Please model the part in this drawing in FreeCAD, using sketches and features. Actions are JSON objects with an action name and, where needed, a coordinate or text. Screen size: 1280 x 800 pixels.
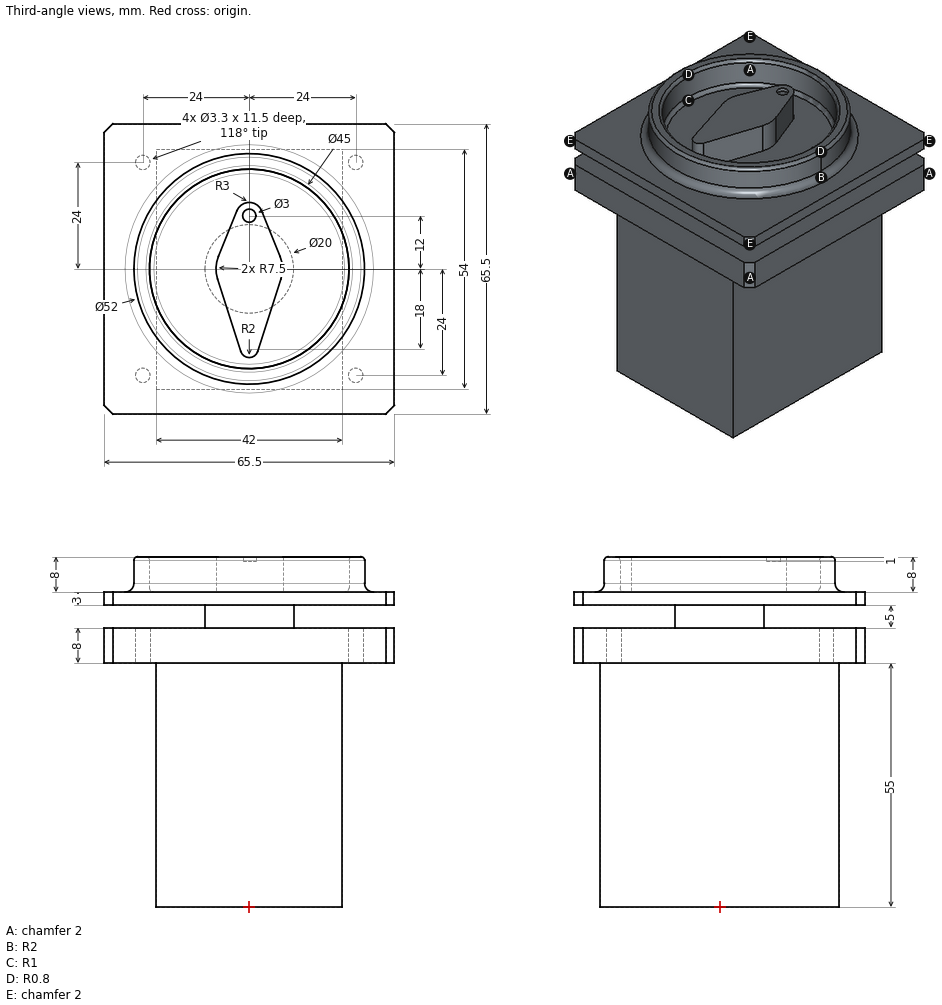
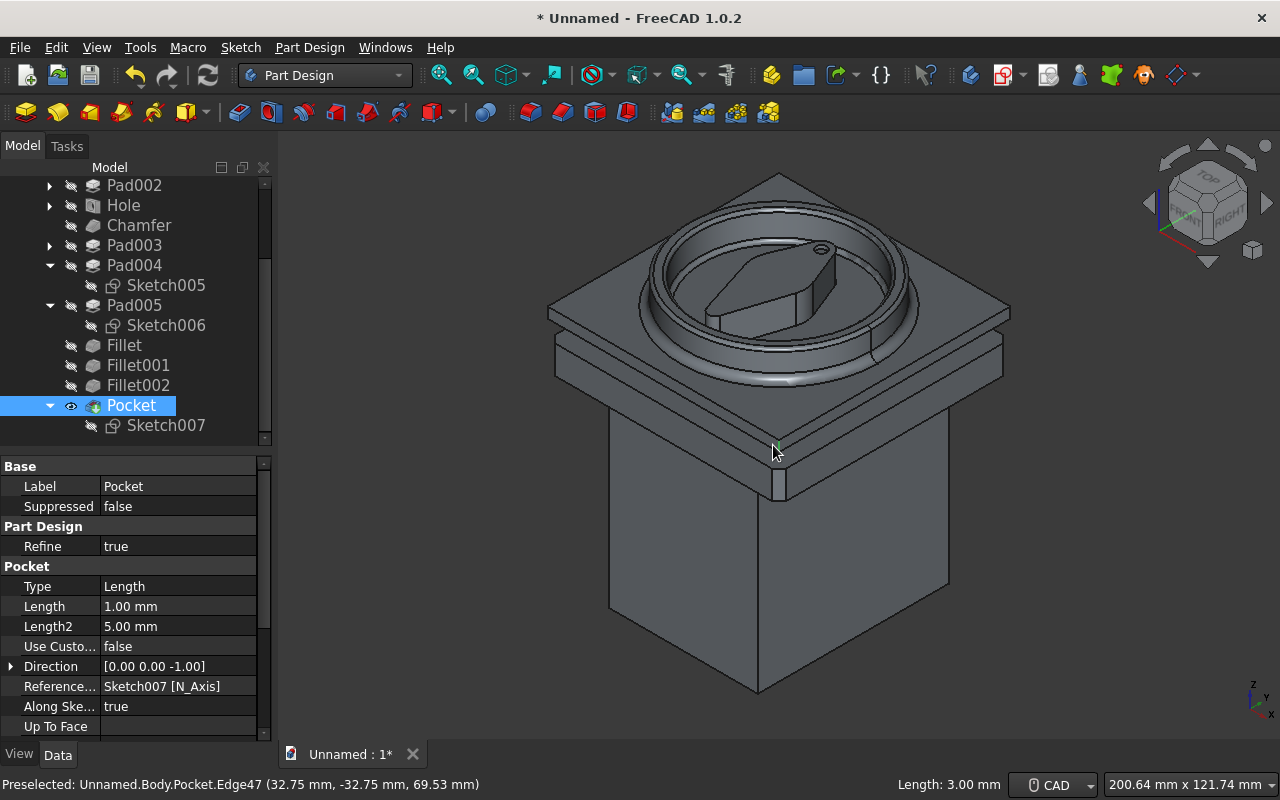
{"action": "scroll", "coordinate": [1010, 312], "scroll_direction": "up", "scroll_amount": 5}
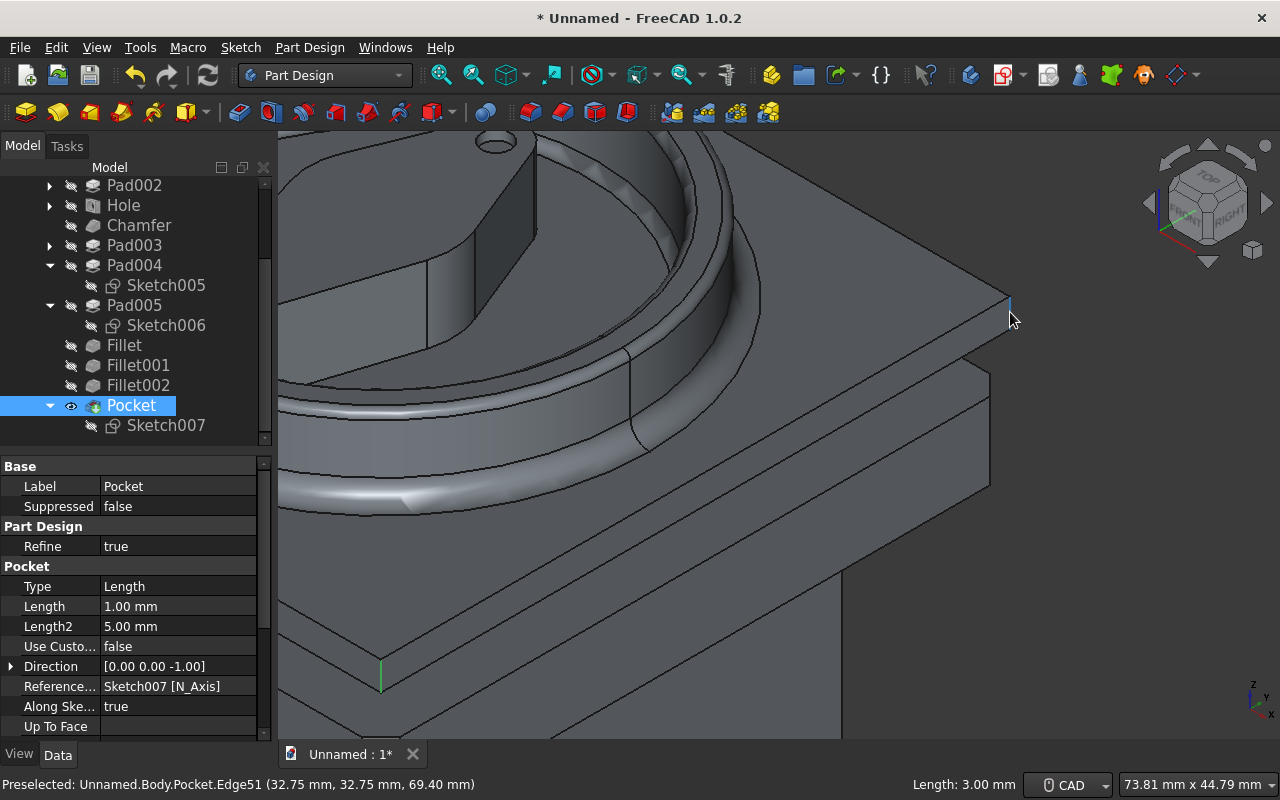
{"action": "left_click", "coordinate": [442, 76]}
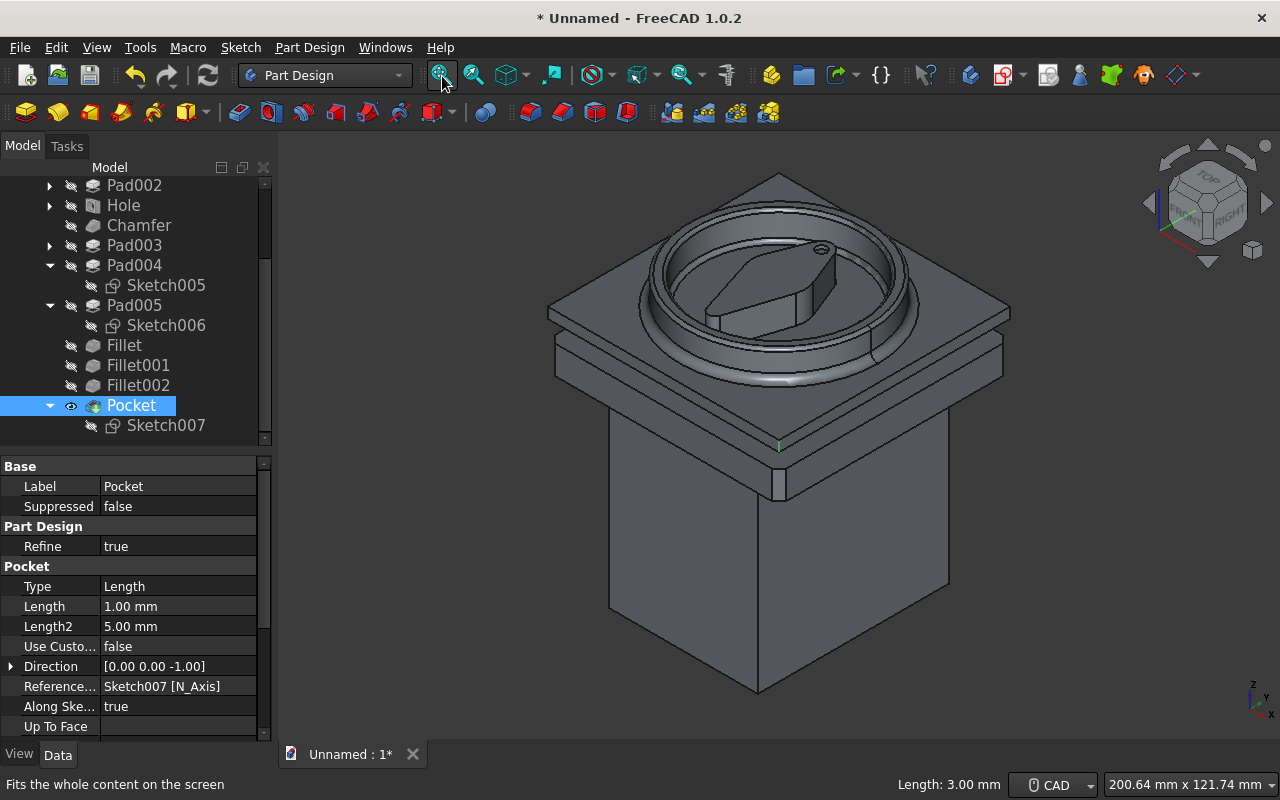
{"action": "key", "text": "2"}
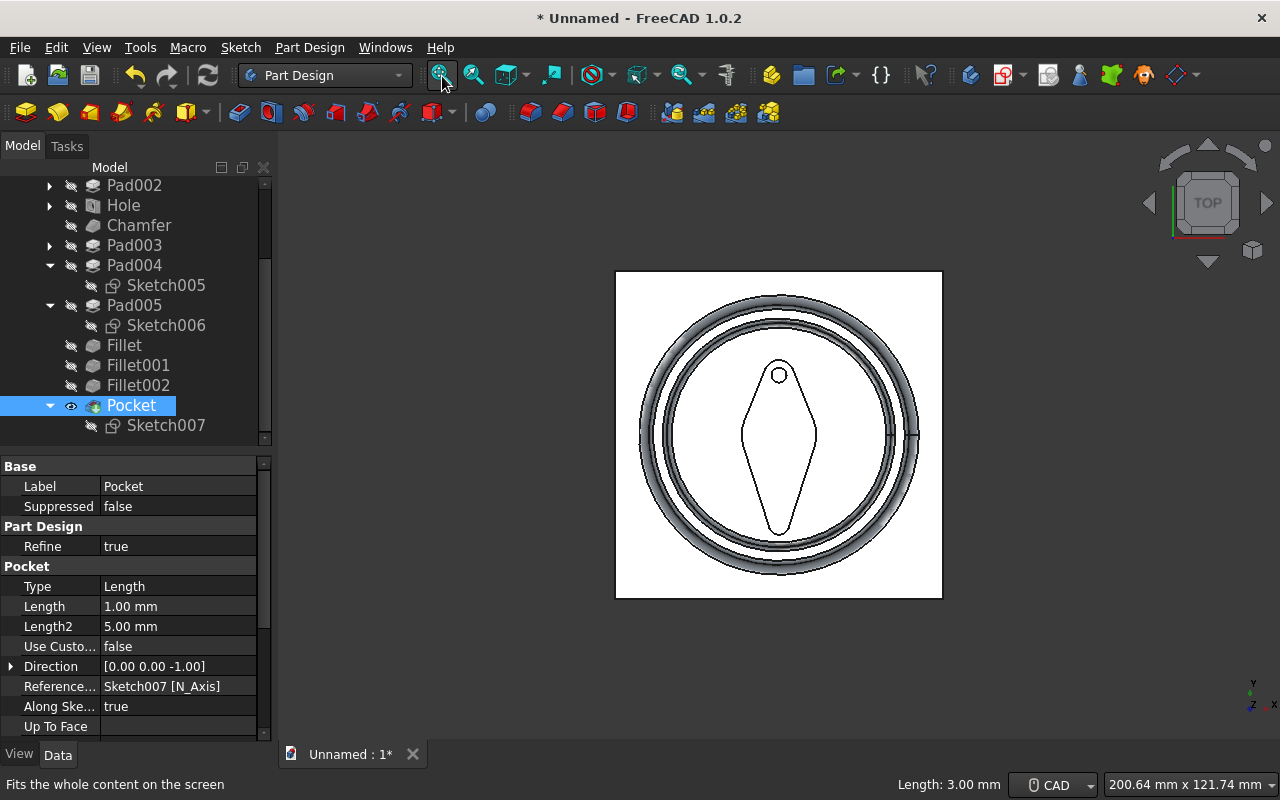
{"action": "scroll", "coordinate": [943, 270], "scroll_direction": "up", "scroll_amount": 5}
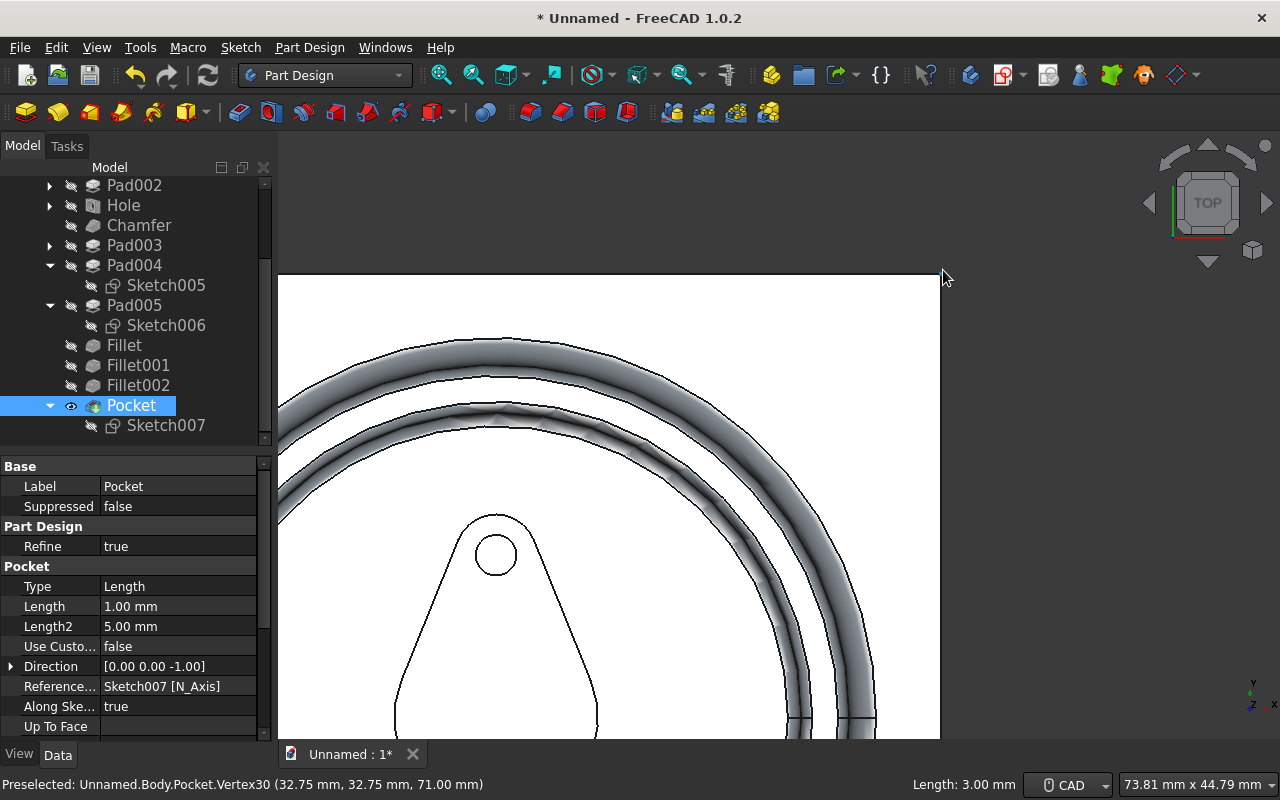
{"action": "left_click", "coordinate": [442, 76]}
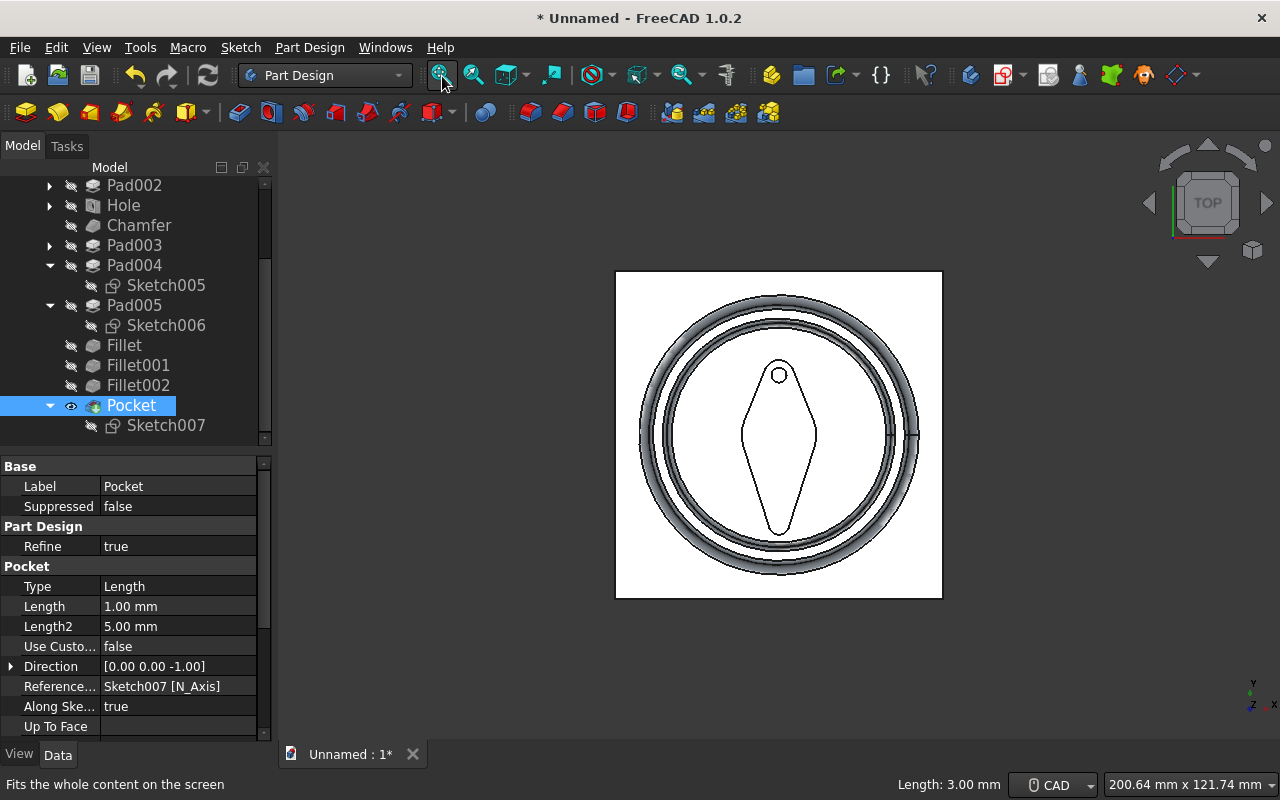
{"action": "key", "text": "0"}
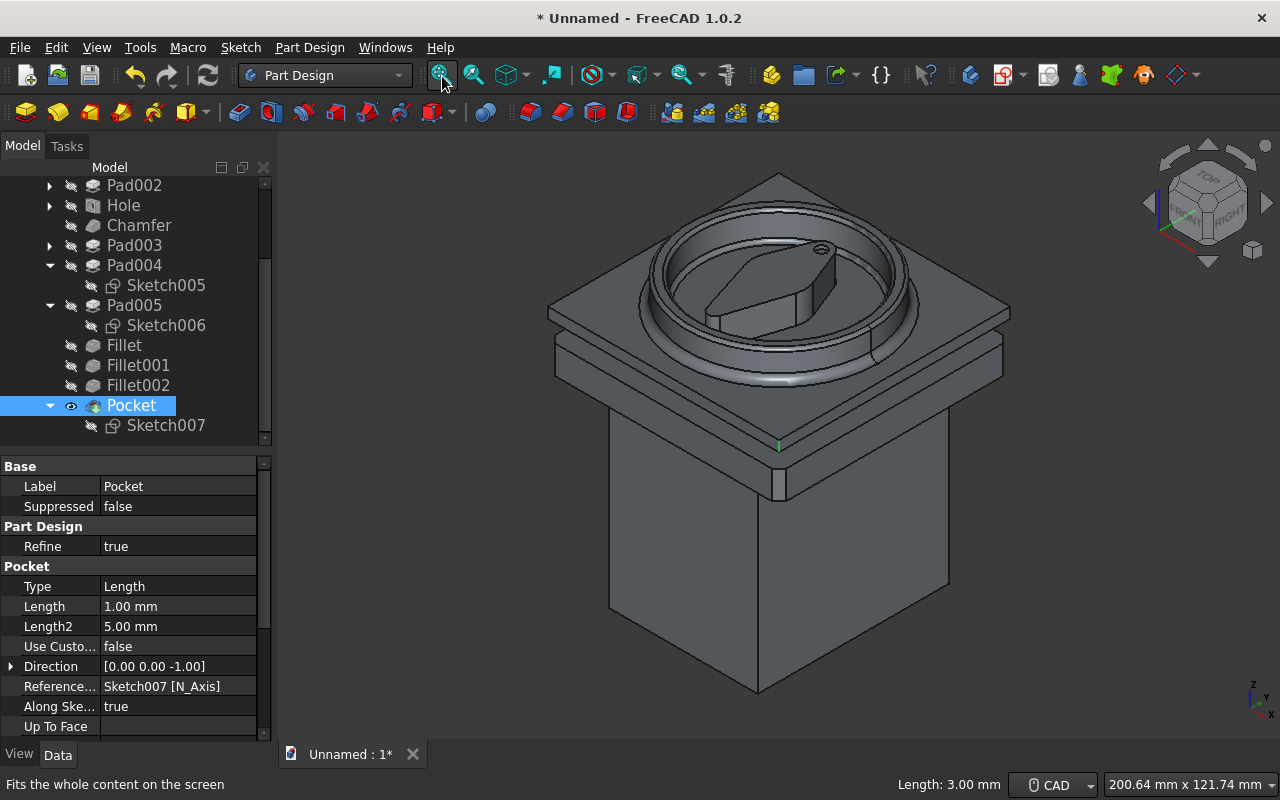
{"action": "scroll", "coordinate": [1010, 312], "scroll_direction": "up", "scroll_amount": 5}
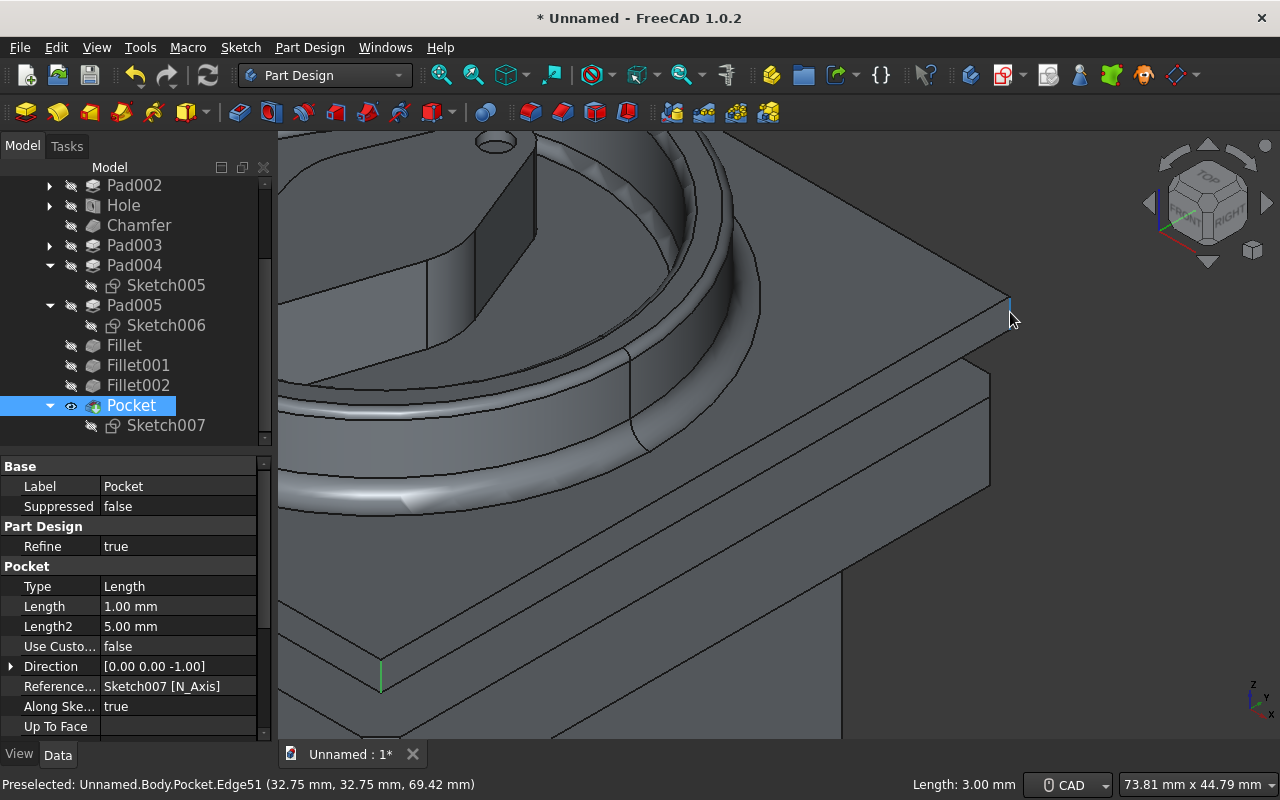
{"action": "left_click", "coordinate": [442, 76]}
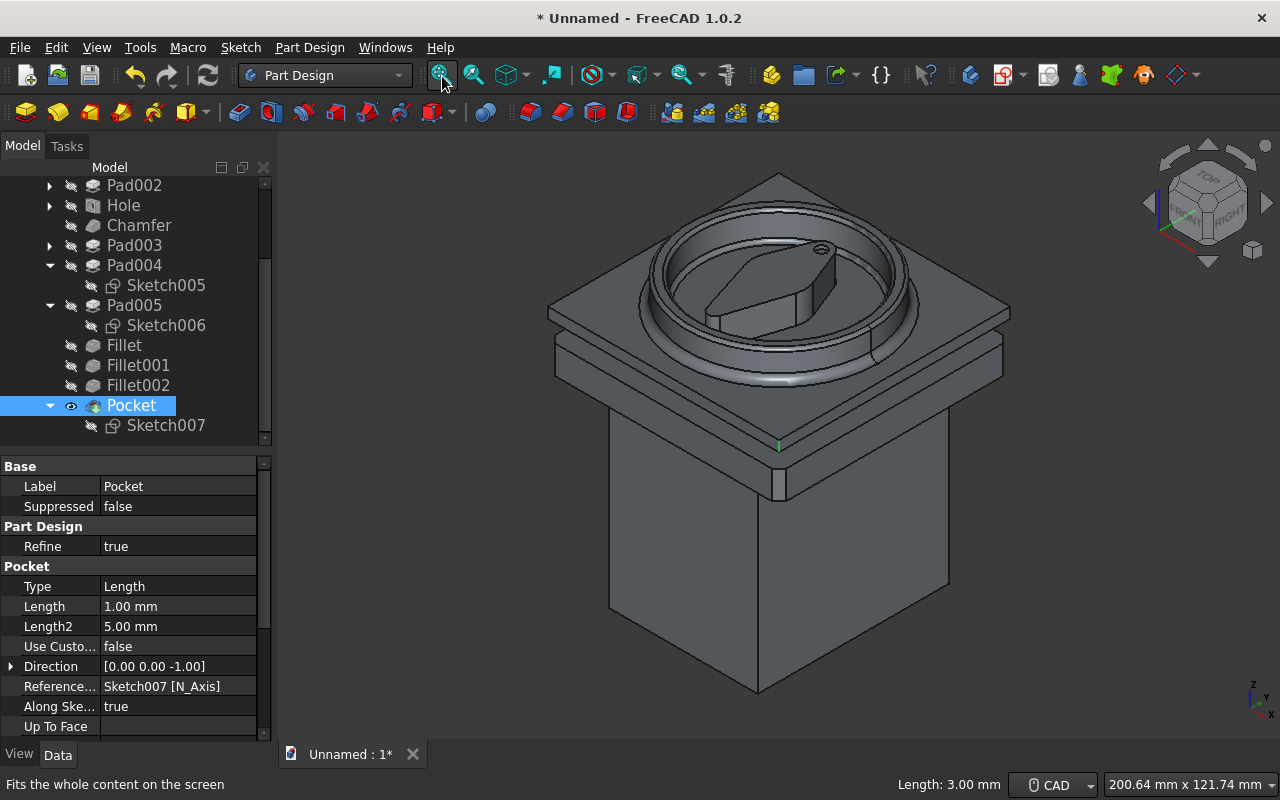
{"action": "key", "text": "1"}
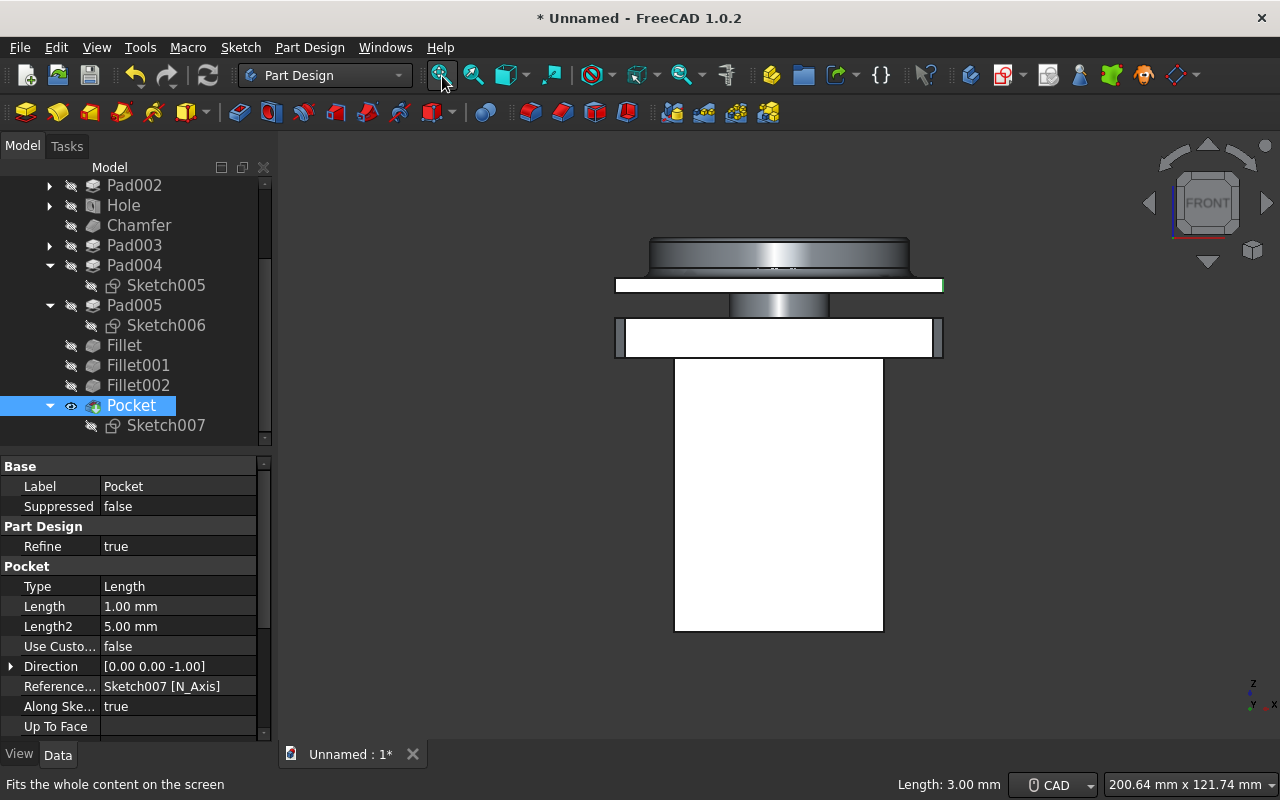
{"action": "left_click", "coordinate": [615, 284], "text": "ctrl"}